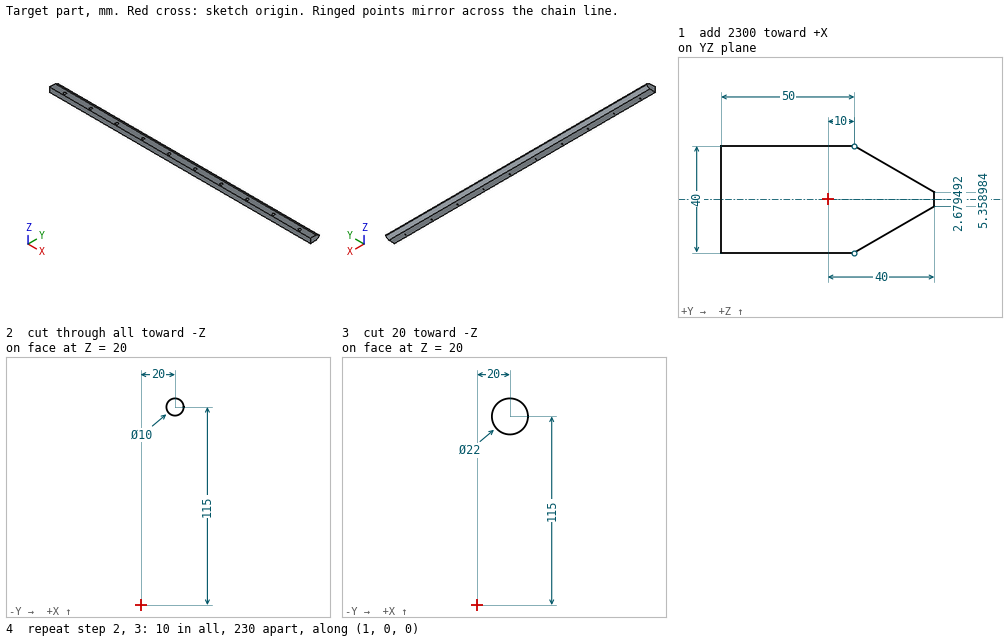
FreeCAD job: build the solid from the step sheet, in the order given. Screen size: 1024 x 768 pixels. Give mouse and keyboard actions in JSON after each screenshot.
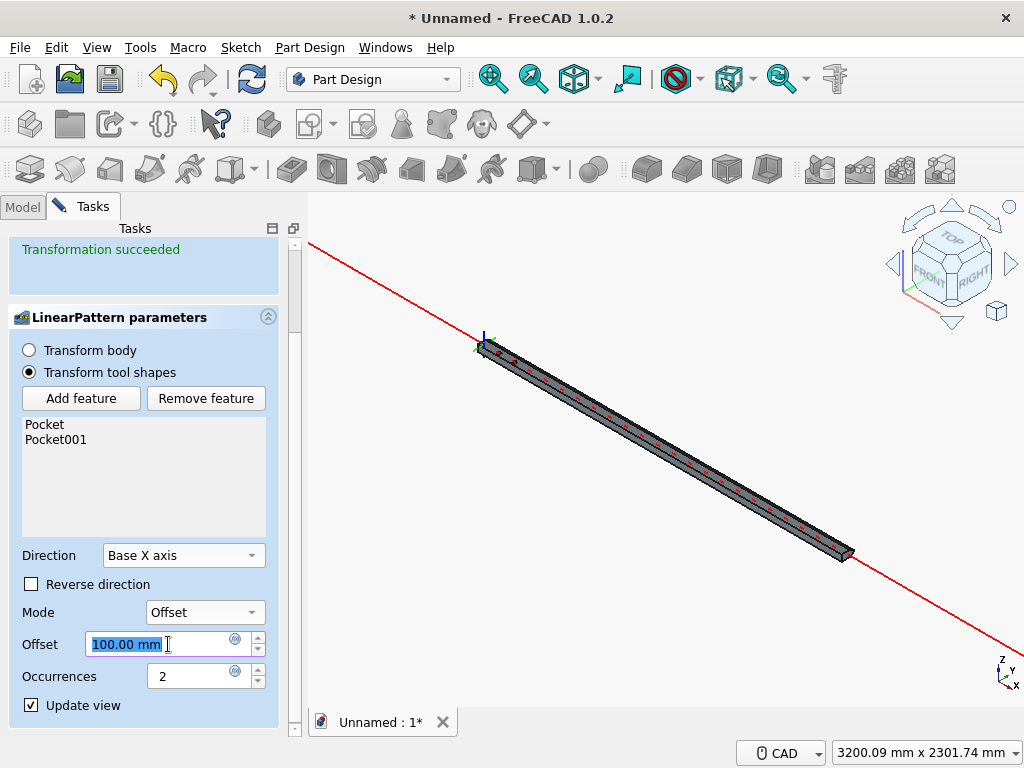
{"action": "type", "text": "230"}
{"action": "key", "text": "Tab"}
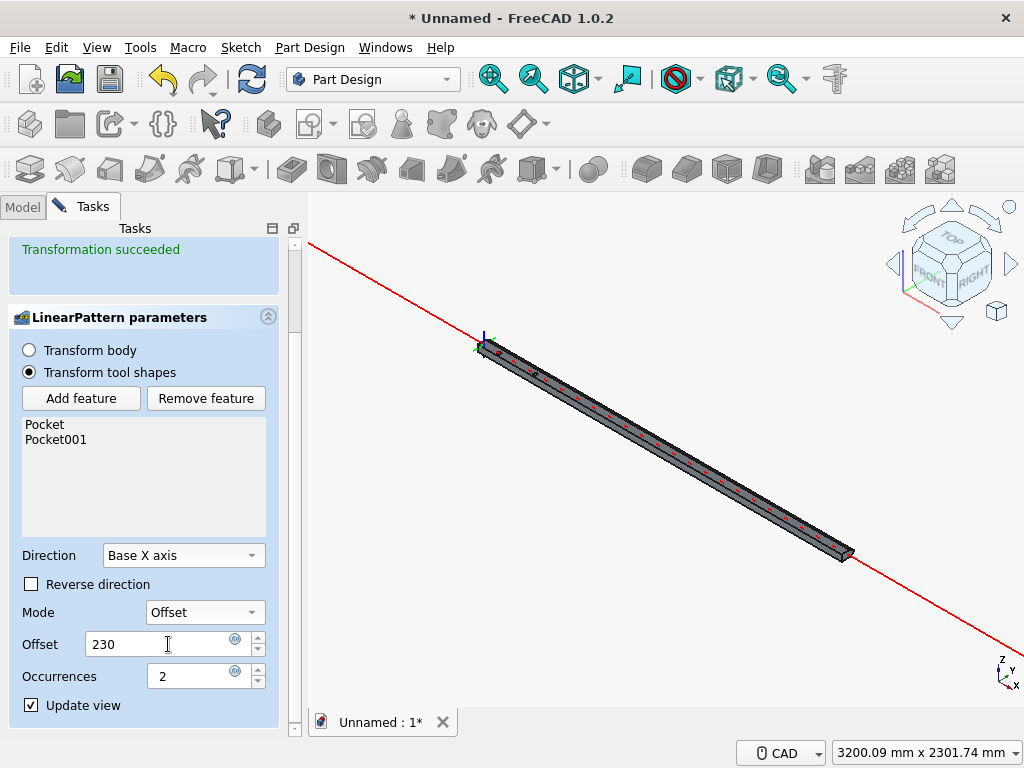
{"action": "triple_click", "coordinate": [198, 676]}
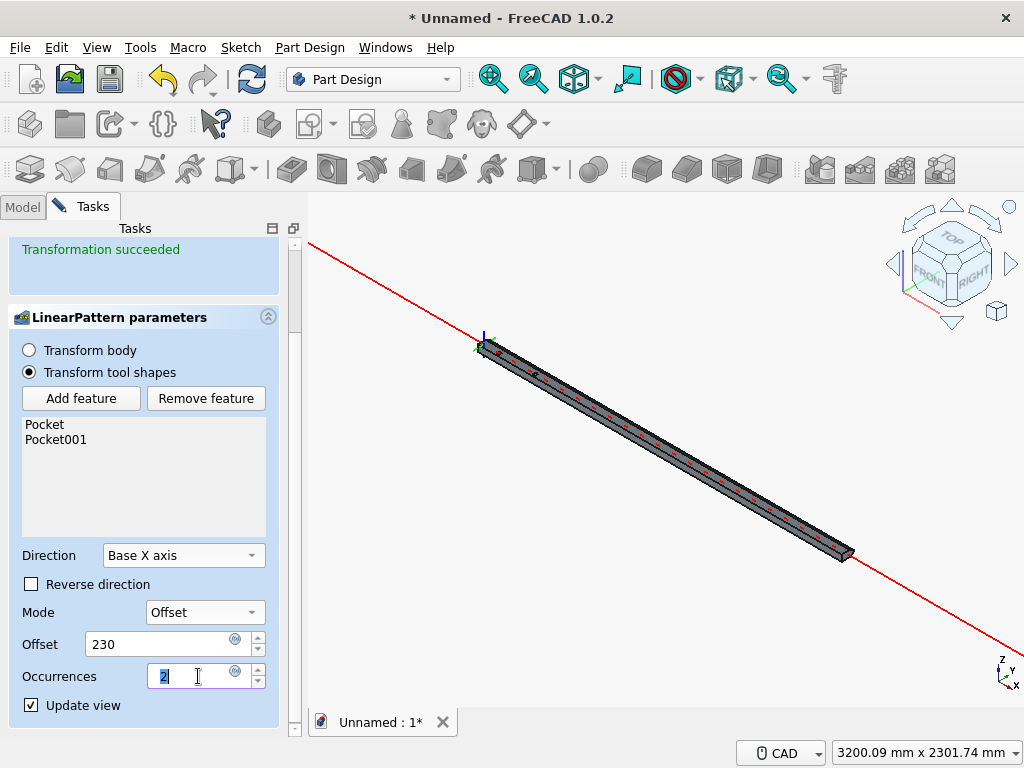
{"action": "type", "text": "10"}
{"action": "key", "text": "Tab"}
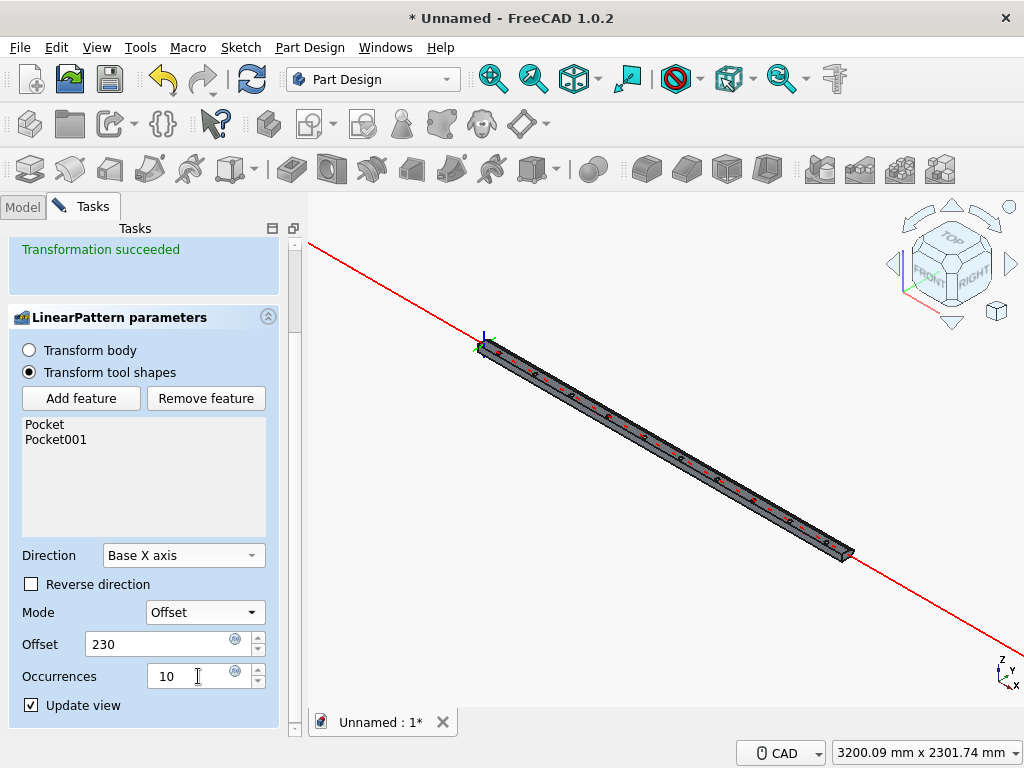
{"action": "scroll", "coordinate": [295, 487], "scroll_direction": "up", "scroll_amount": 3}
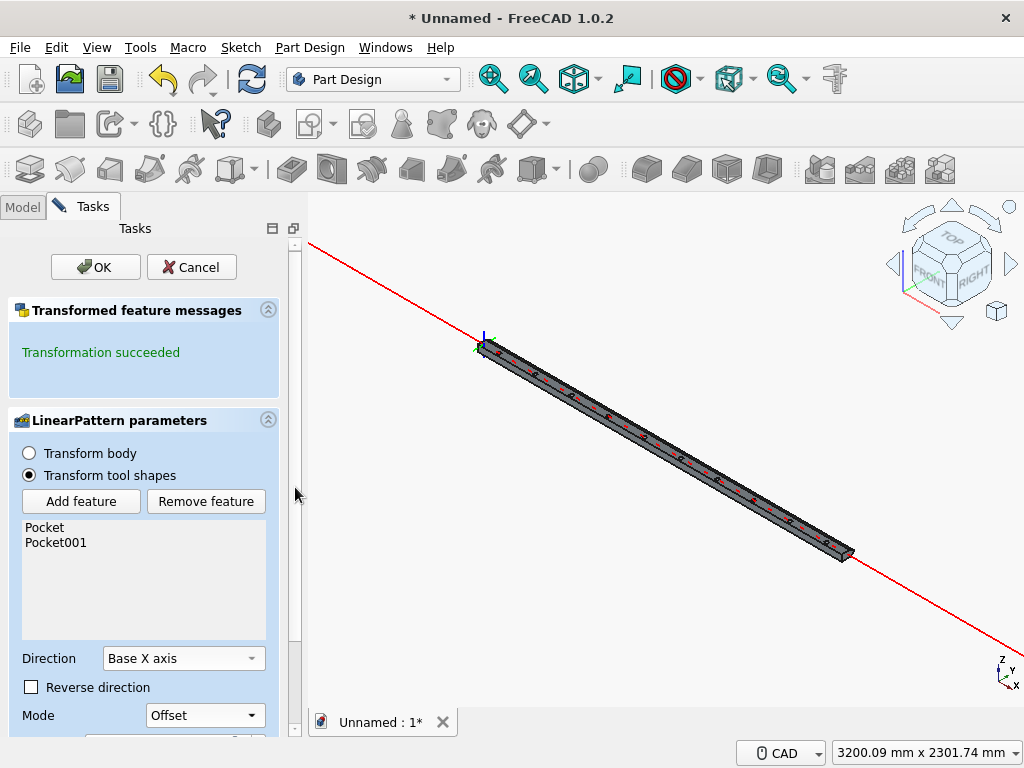
{"action": "left_click", "coordinate": [96, 267]}